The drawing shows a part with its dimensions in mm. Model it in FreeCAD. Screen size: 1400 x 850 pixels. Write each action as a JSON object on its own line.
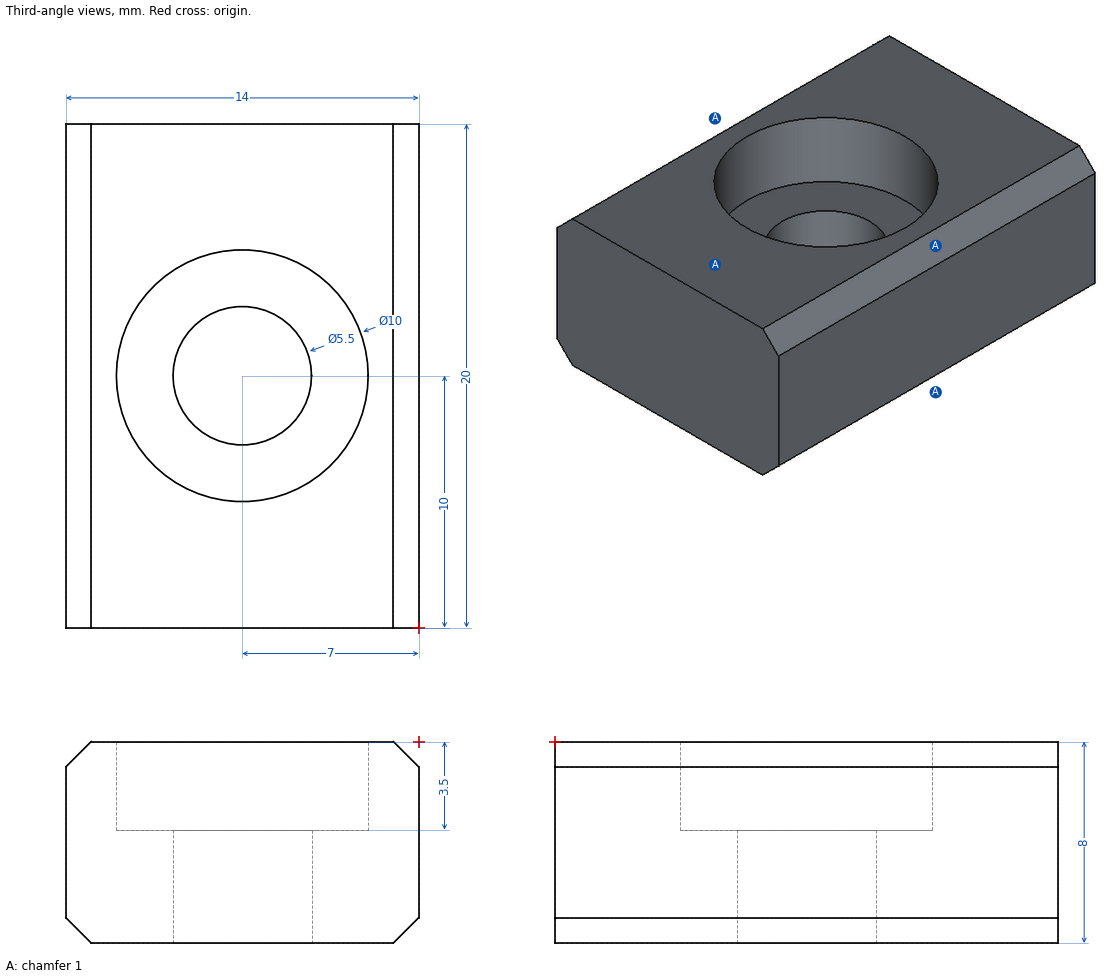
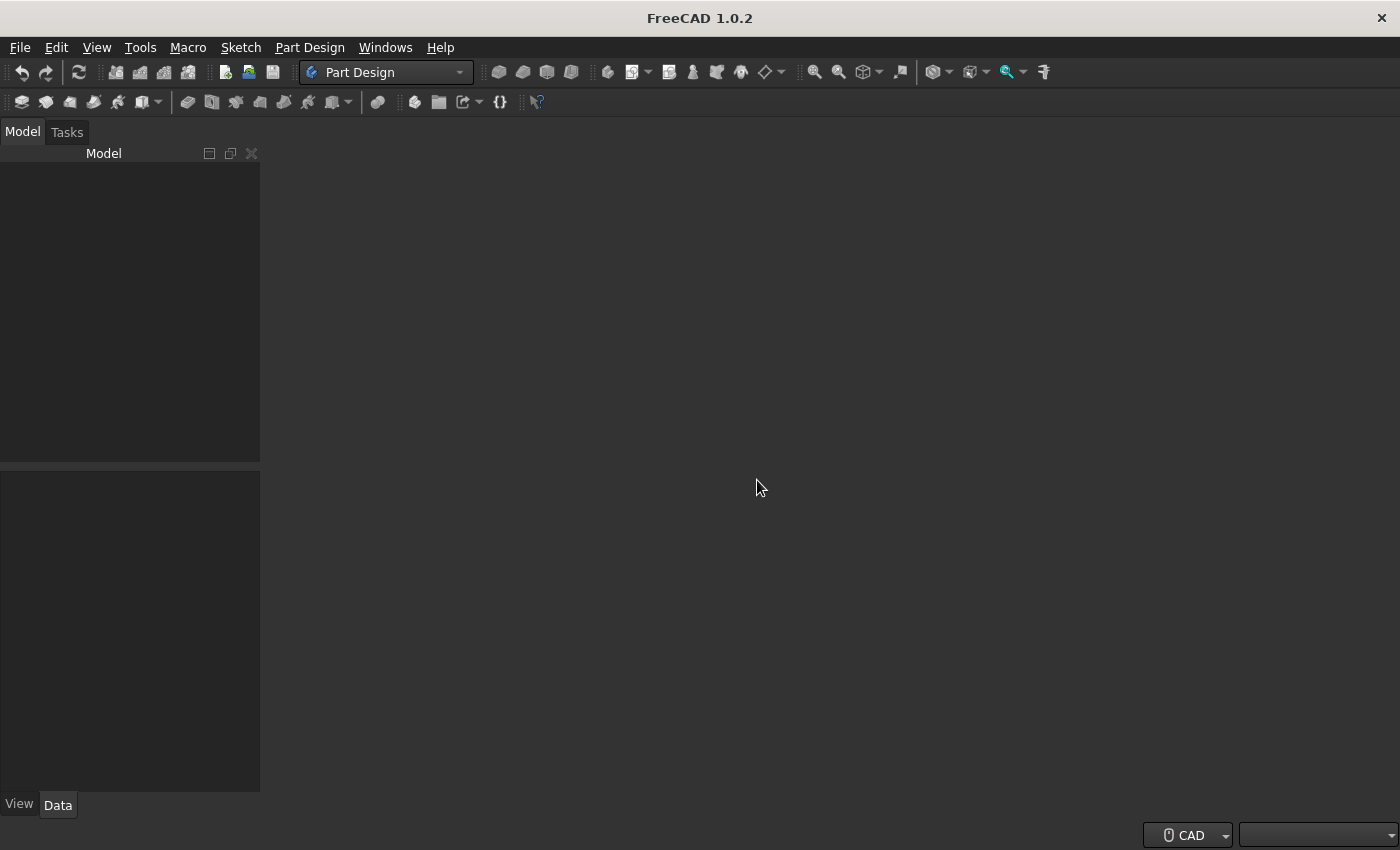
{"action": "key", "text": "ctrl+n"}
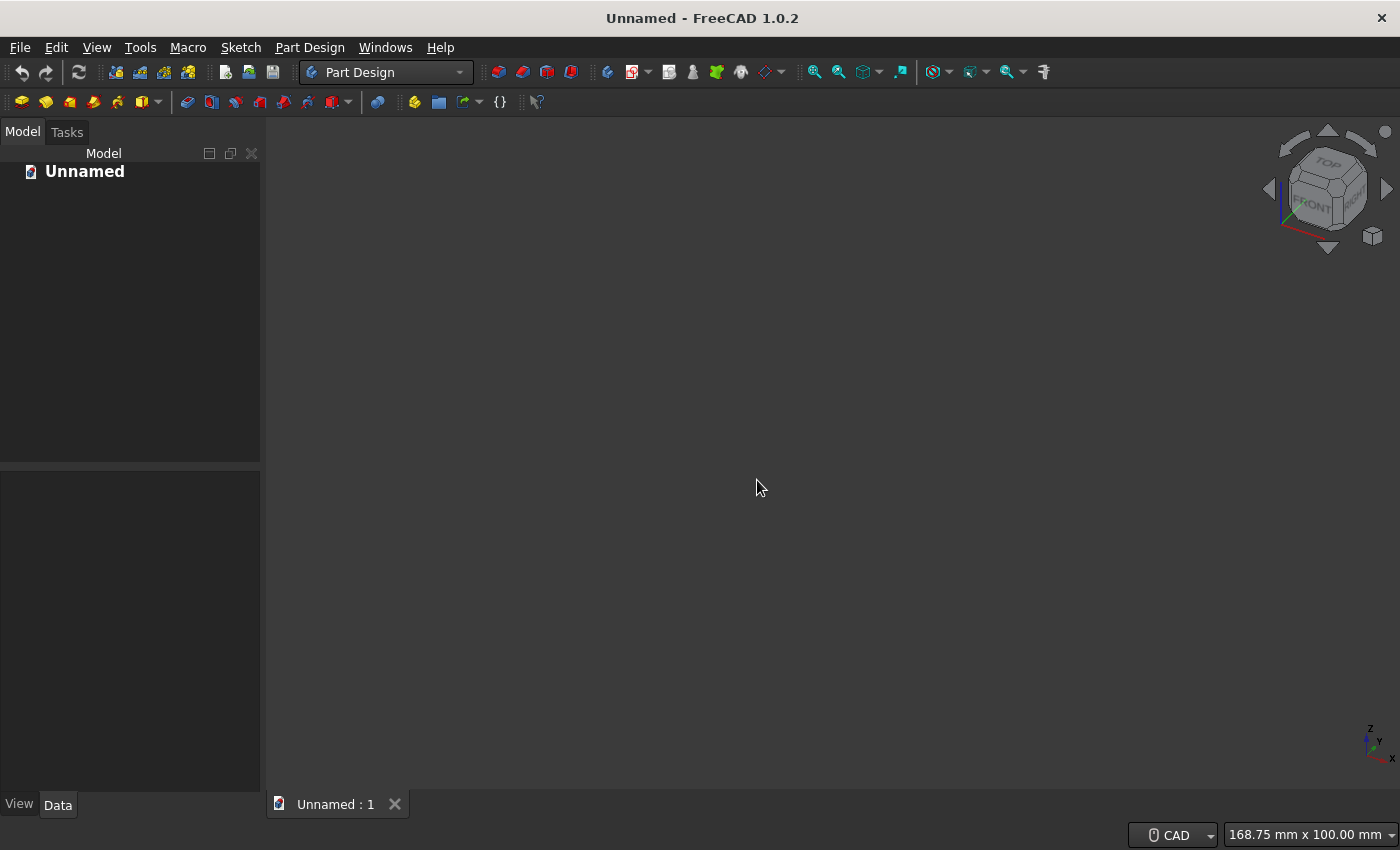
{"action": "left_click", "coordinate": [632, 72]}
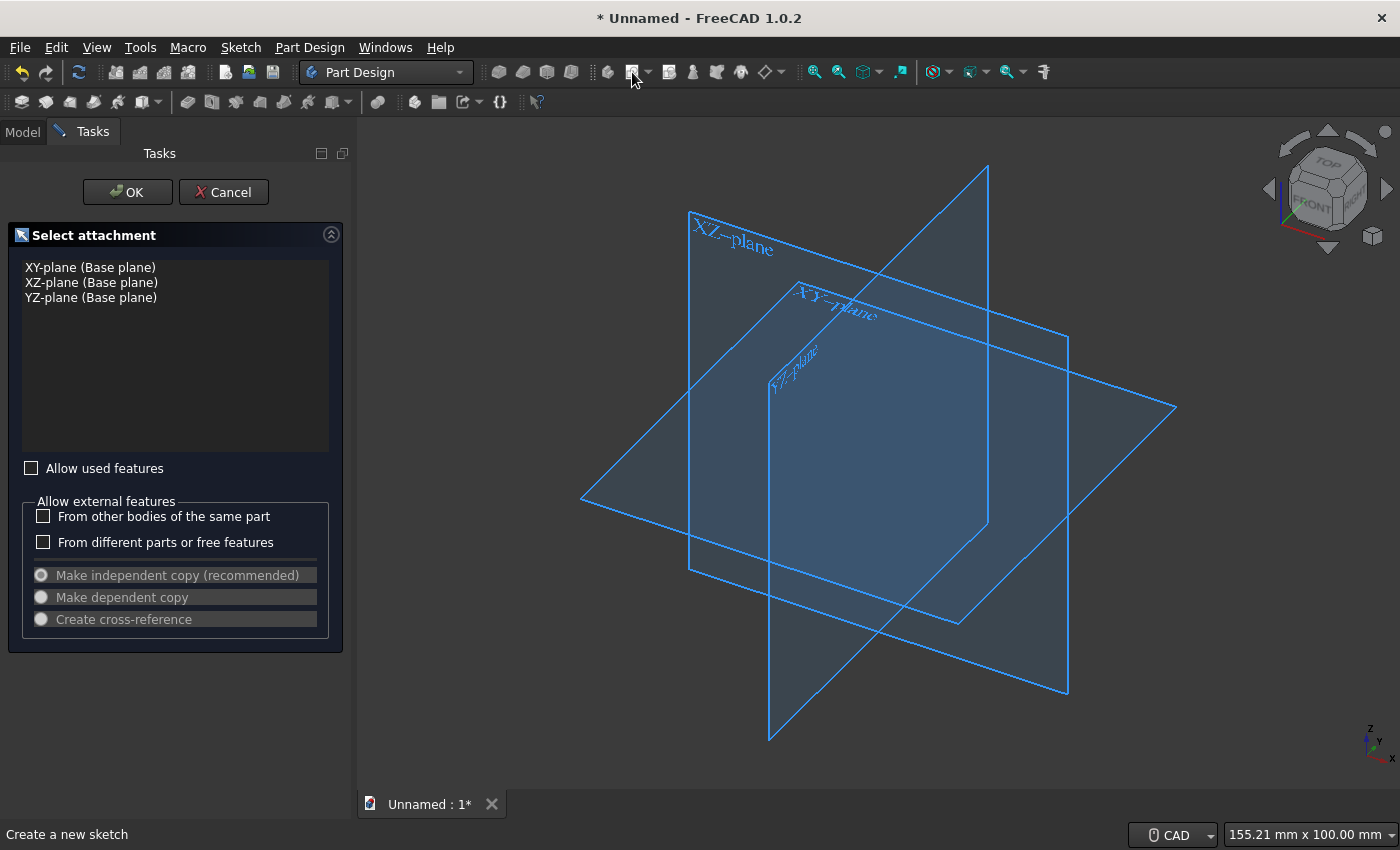
{"action": "left_click", "coordinate": [82, 268]}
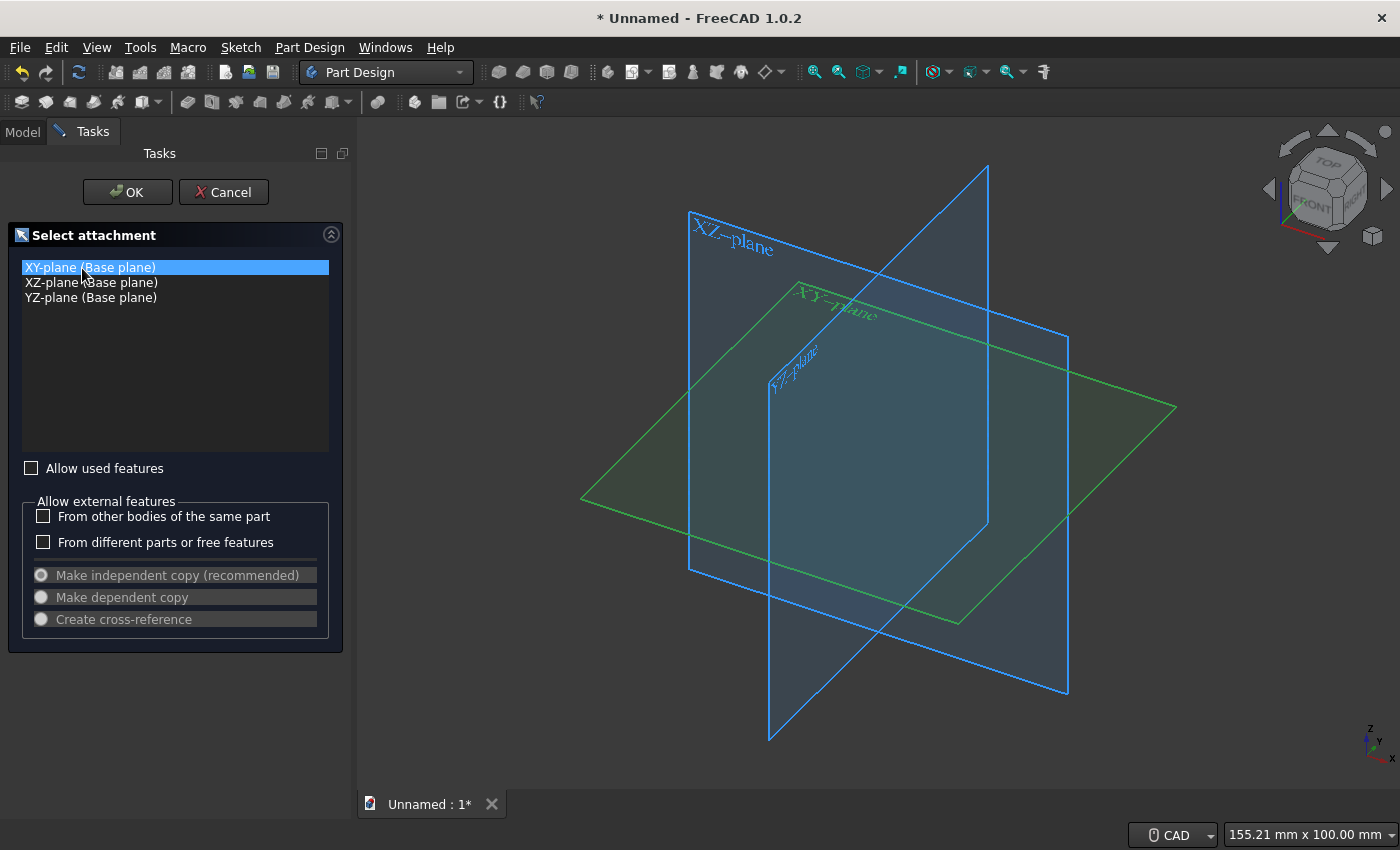
{"action": "left_click", "coordinate": [128, 192]}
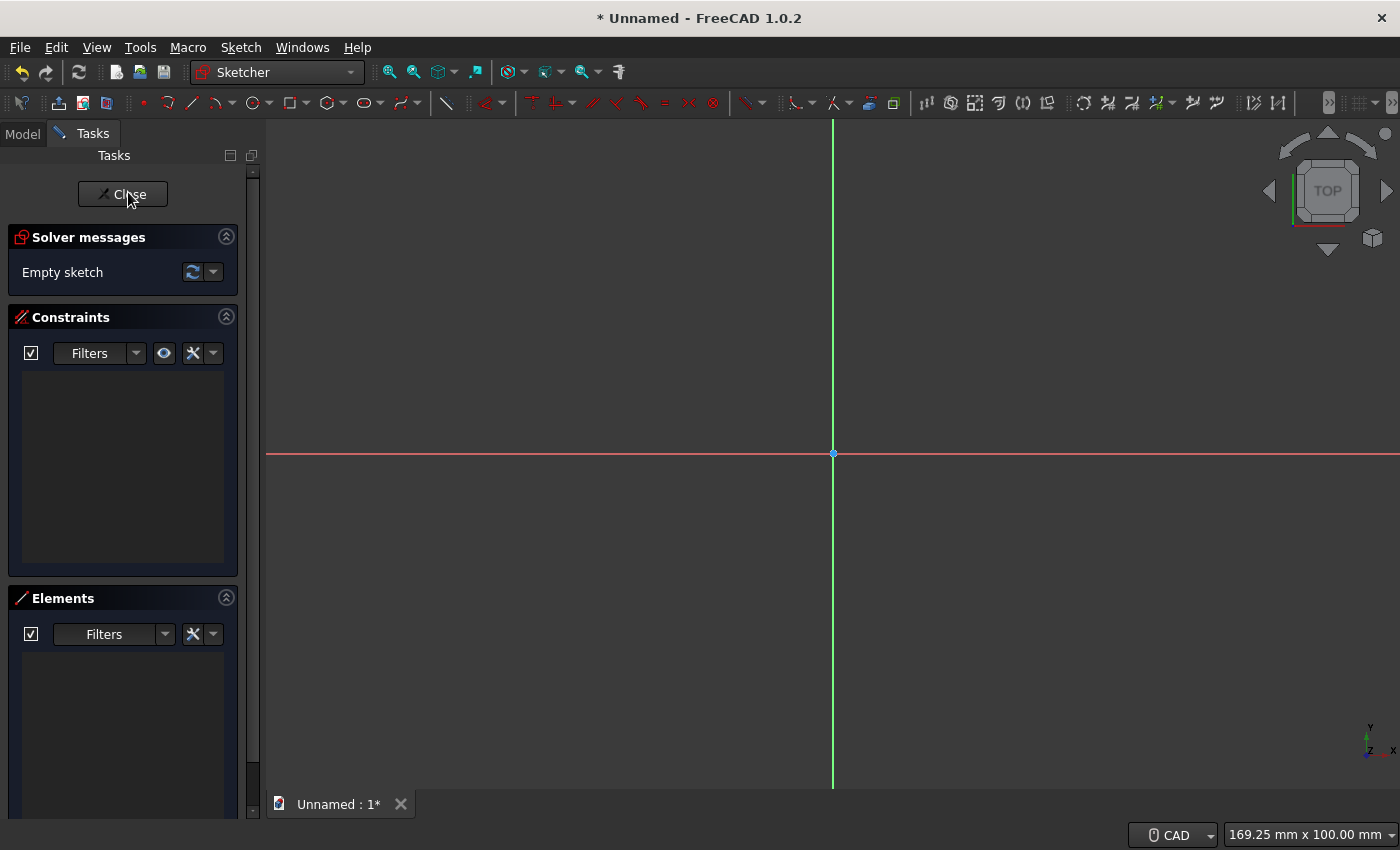
{"action": "scroll", "coordinate": [795, 358], "scroll_direction": "up", "scroll_amount": 6}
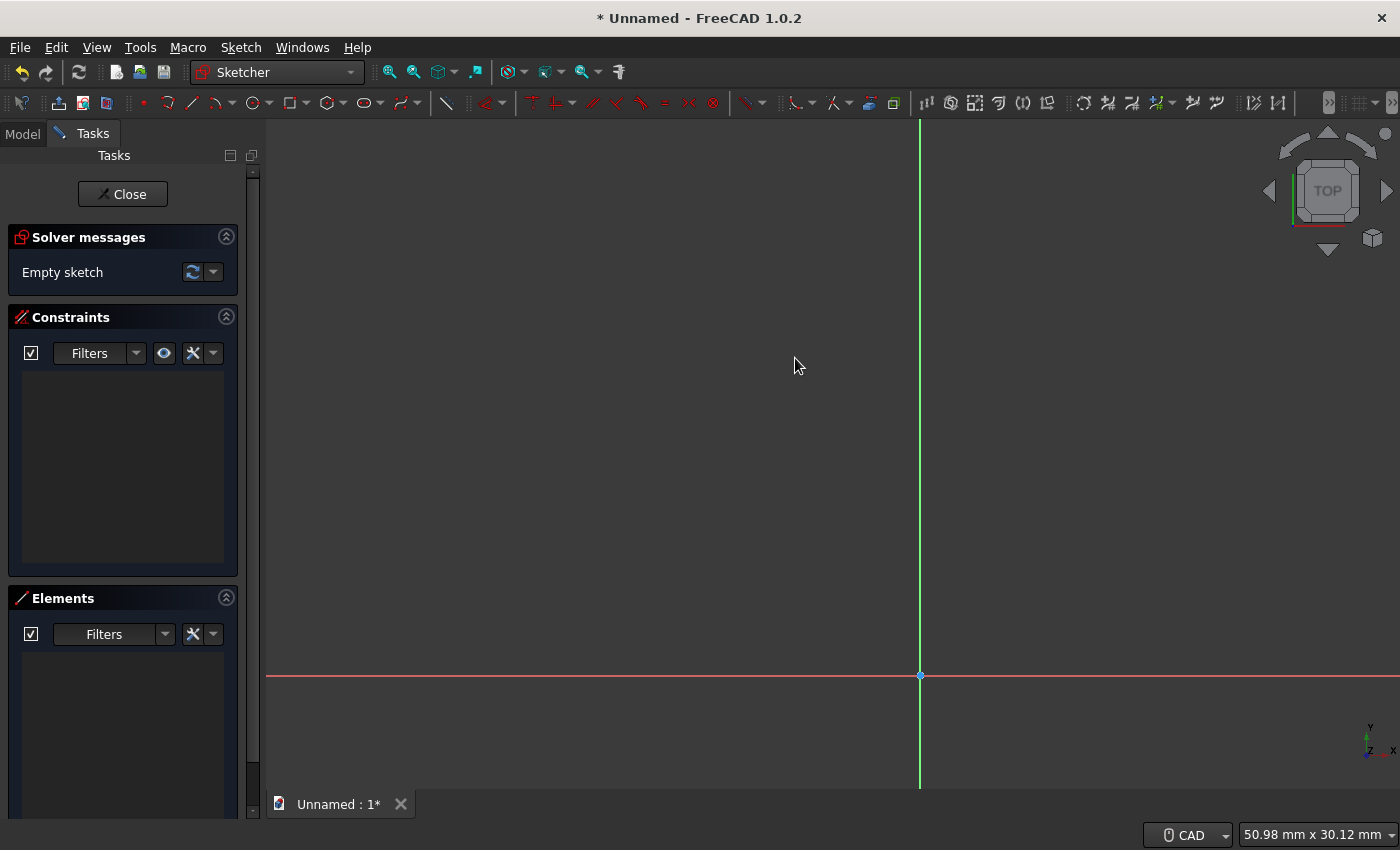
{"action": "key", "text": "g r"}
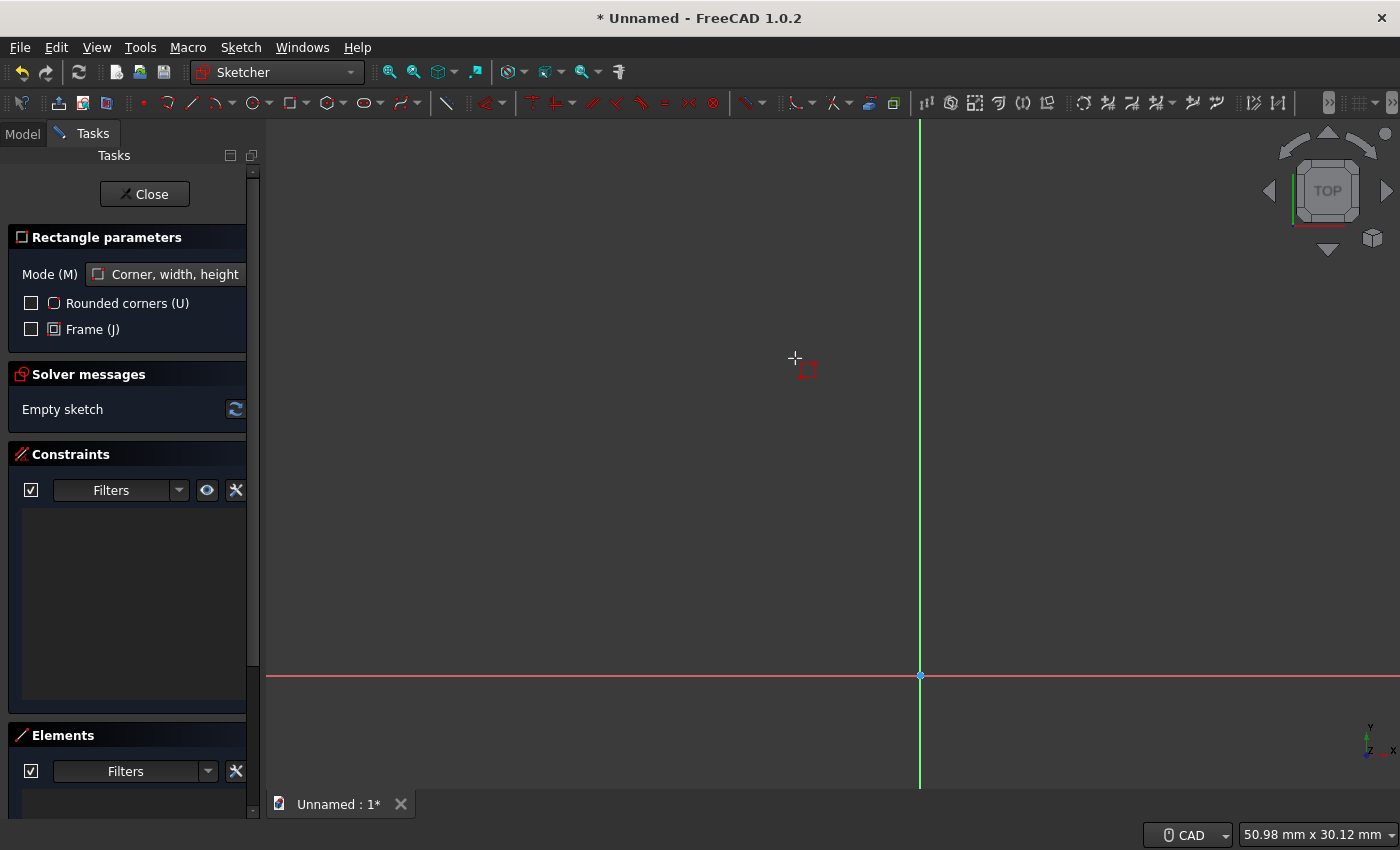
{"action": "left_click", "coordinate": [920, 676]}
{"action": "left_click", "coordinate": [609, 231]}
{"action": "key", "text": "Escape"}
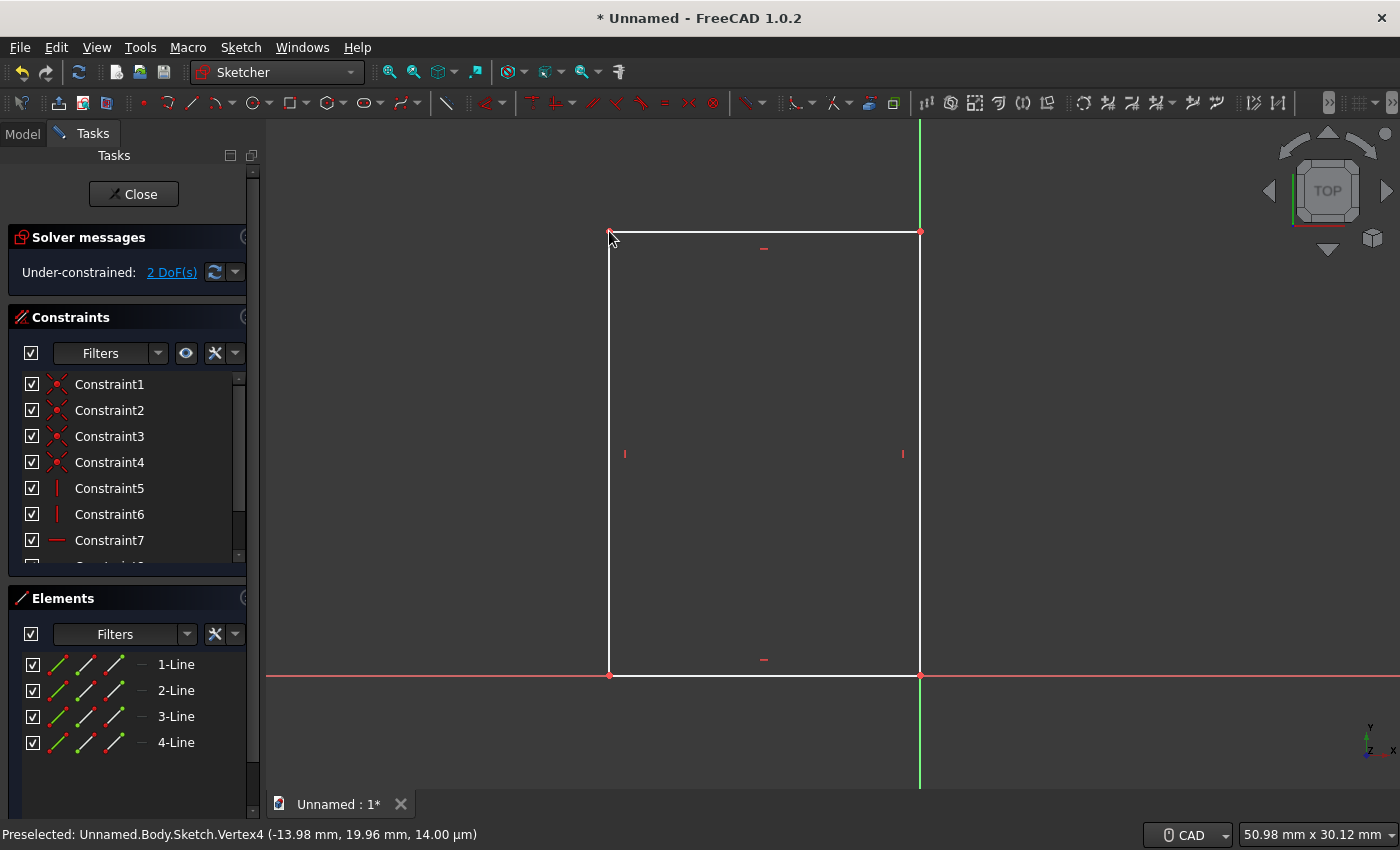
{"action": "key", "text": "d"}